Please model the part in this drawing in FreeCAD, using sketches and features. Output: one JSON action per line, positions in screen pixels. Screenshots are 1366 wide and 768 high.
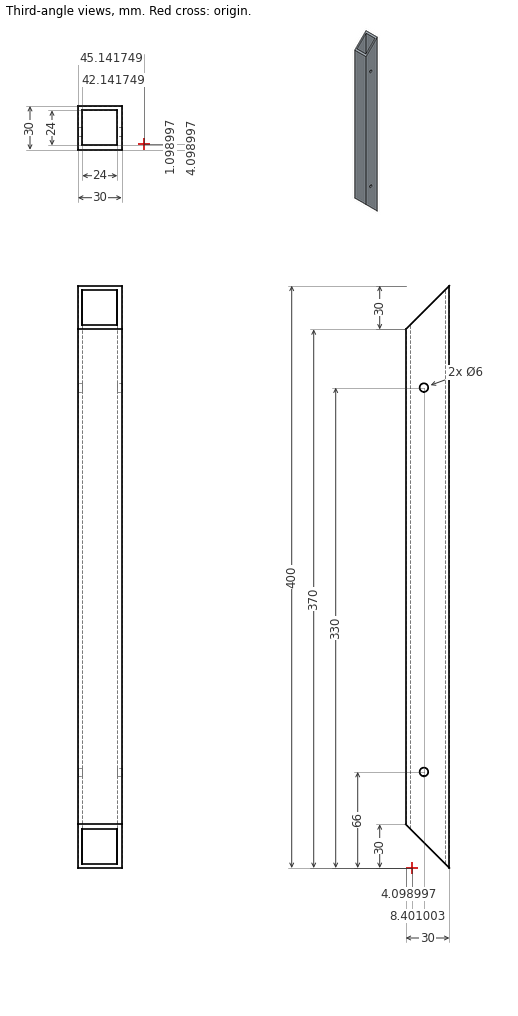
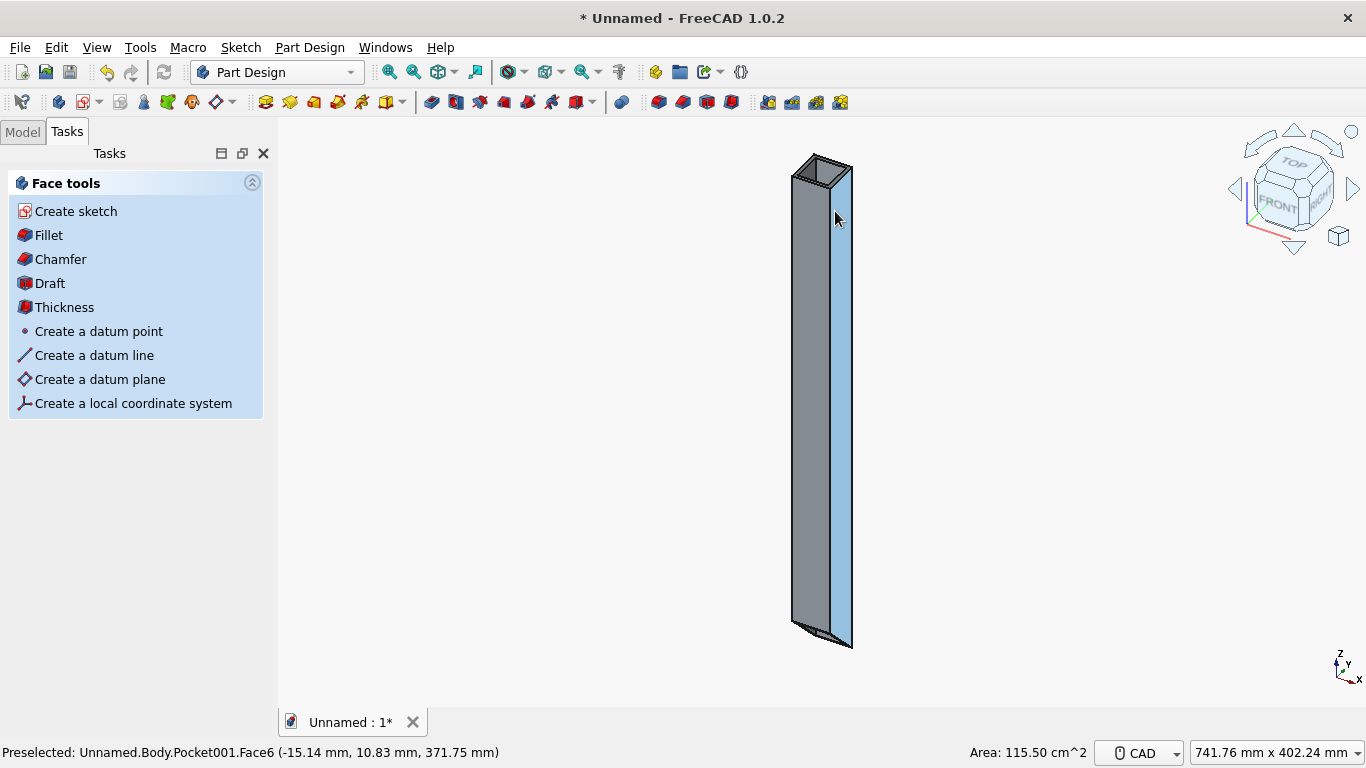
{"action": "left_click", "coordinate": [84, 102]}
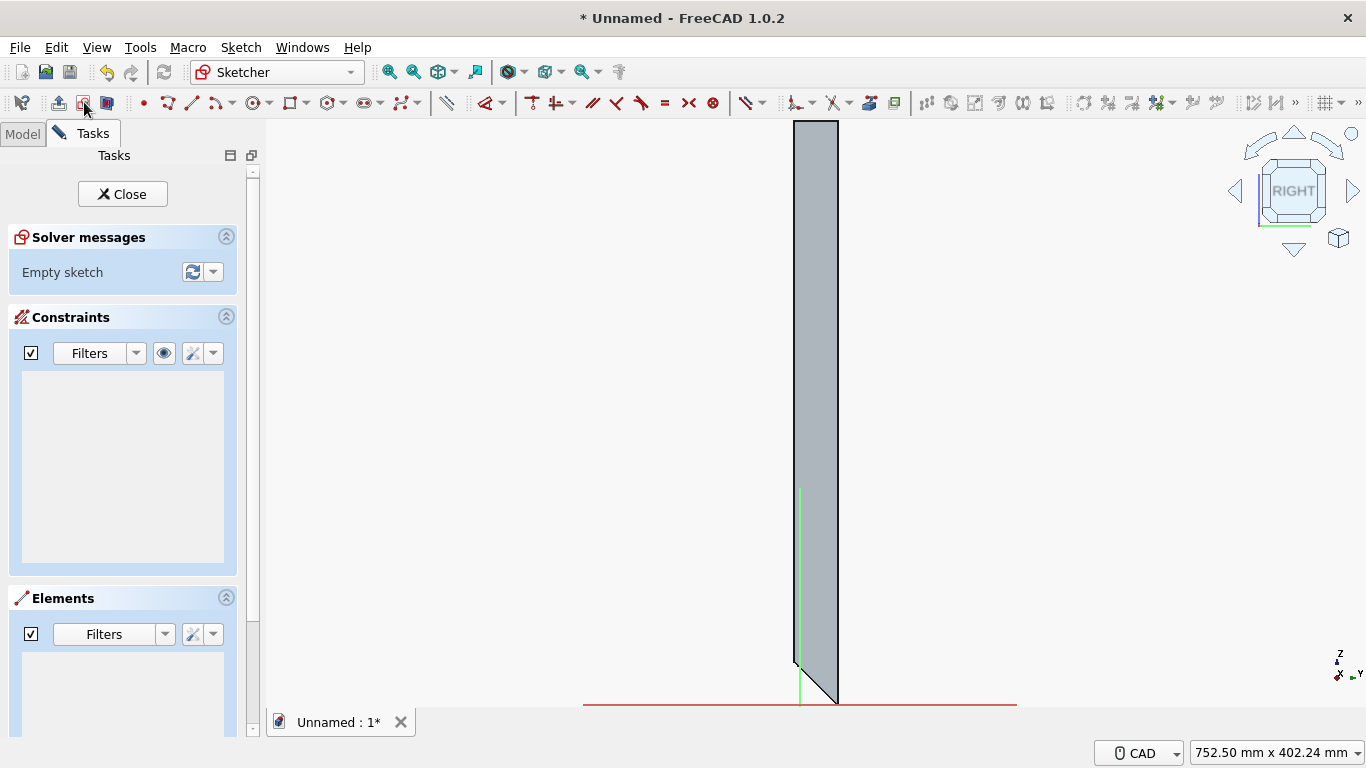
{"action": "scroll", "coordinate": [748, 413], "scroll_direction": "down", "scroll_amount": 5}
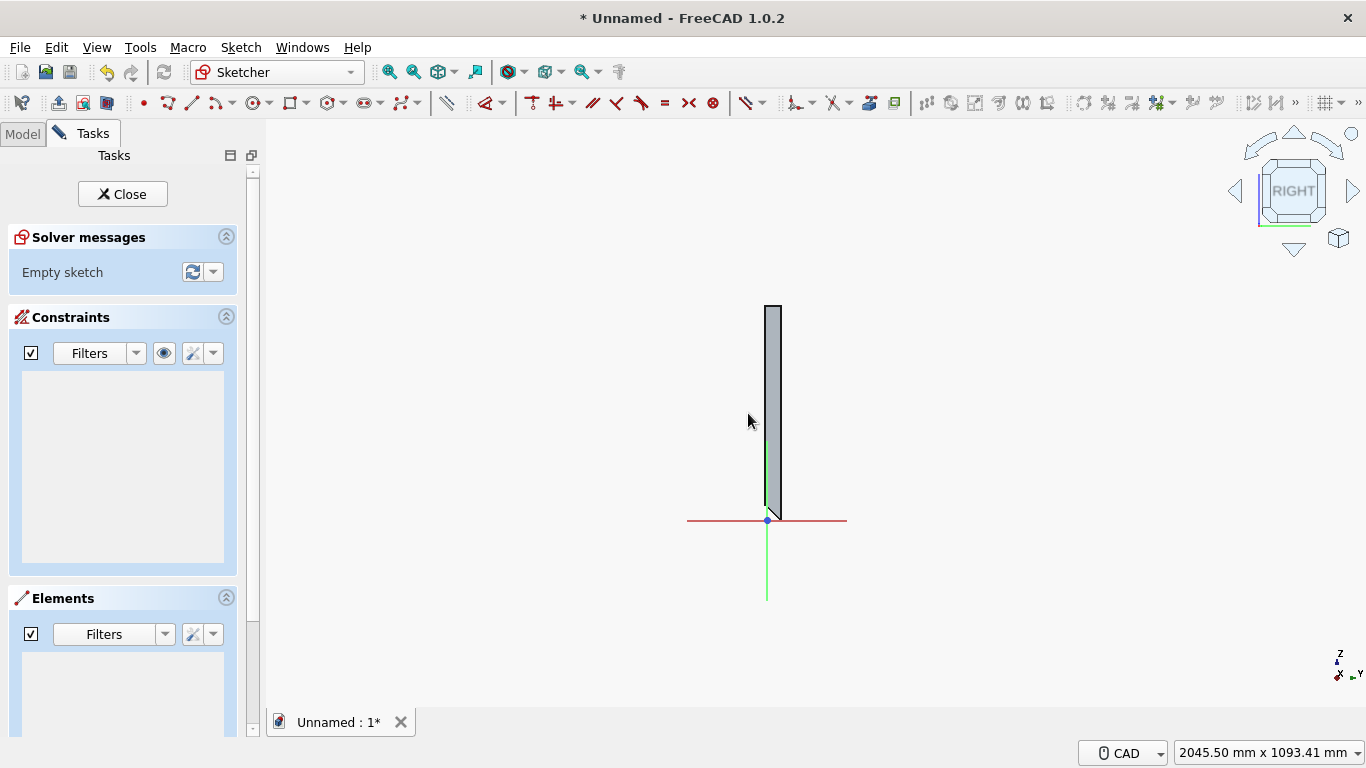
{"action": "scroll", "coordinate": [775, 309], "scroll_direction": "up", "scroll_amount": 15}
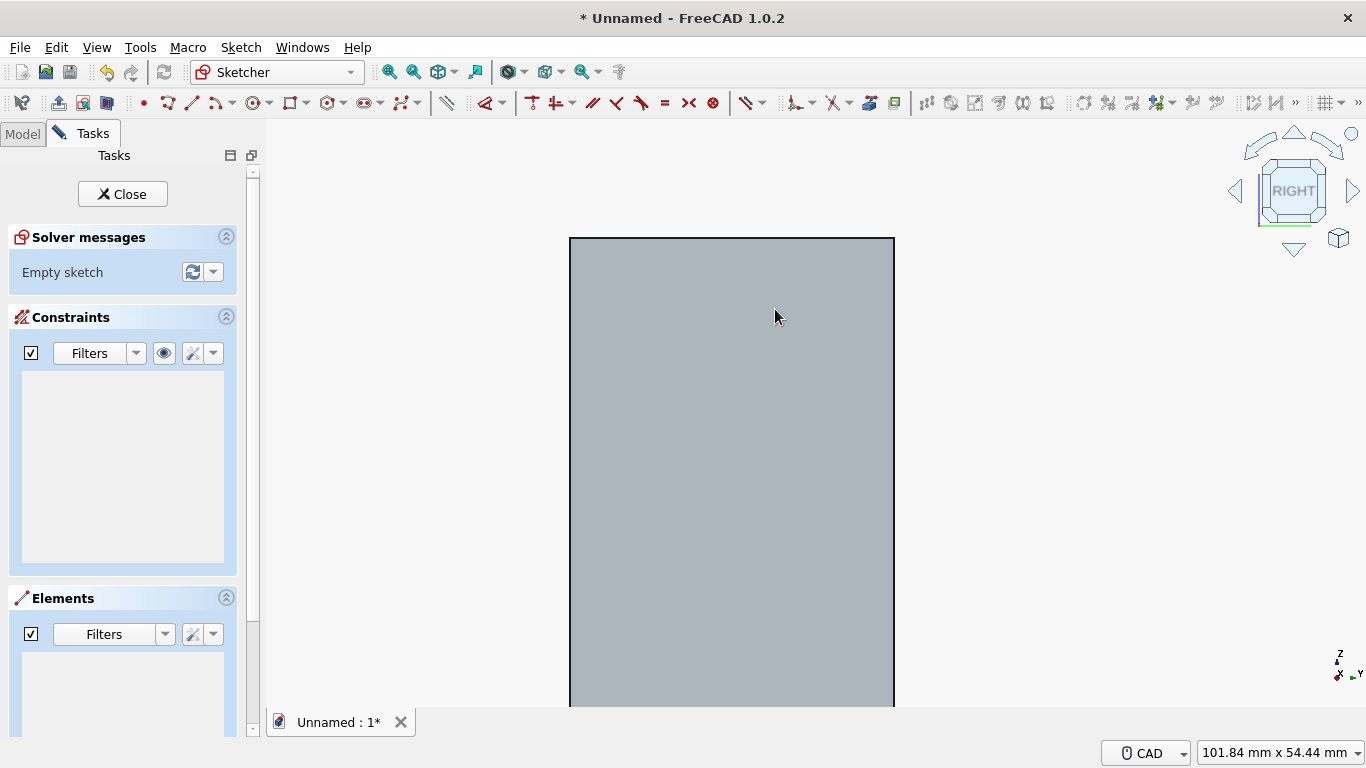
{"action": "left_click", "coordinate": [168, 104]}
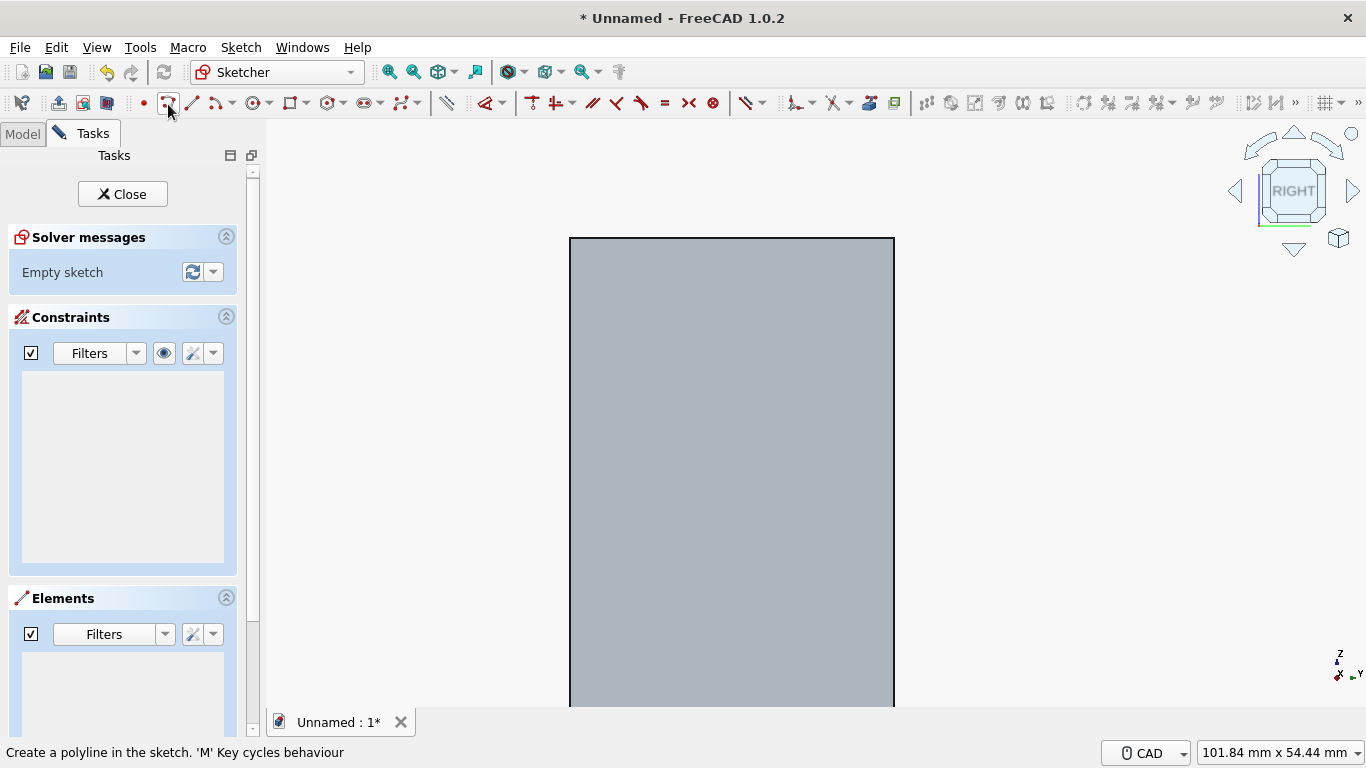
{"action": "left_click", "coordinate": [570, 562]}
{"action": "left_click", "coordinate": [894, 238]}
{"action": "left_click", "coordinate": [570, 238]}
{"action": "left_click", "coordinate": [570, 563]}
{"action": "key", "text": "Escape"}
{"action": "key", "text": "Escape"}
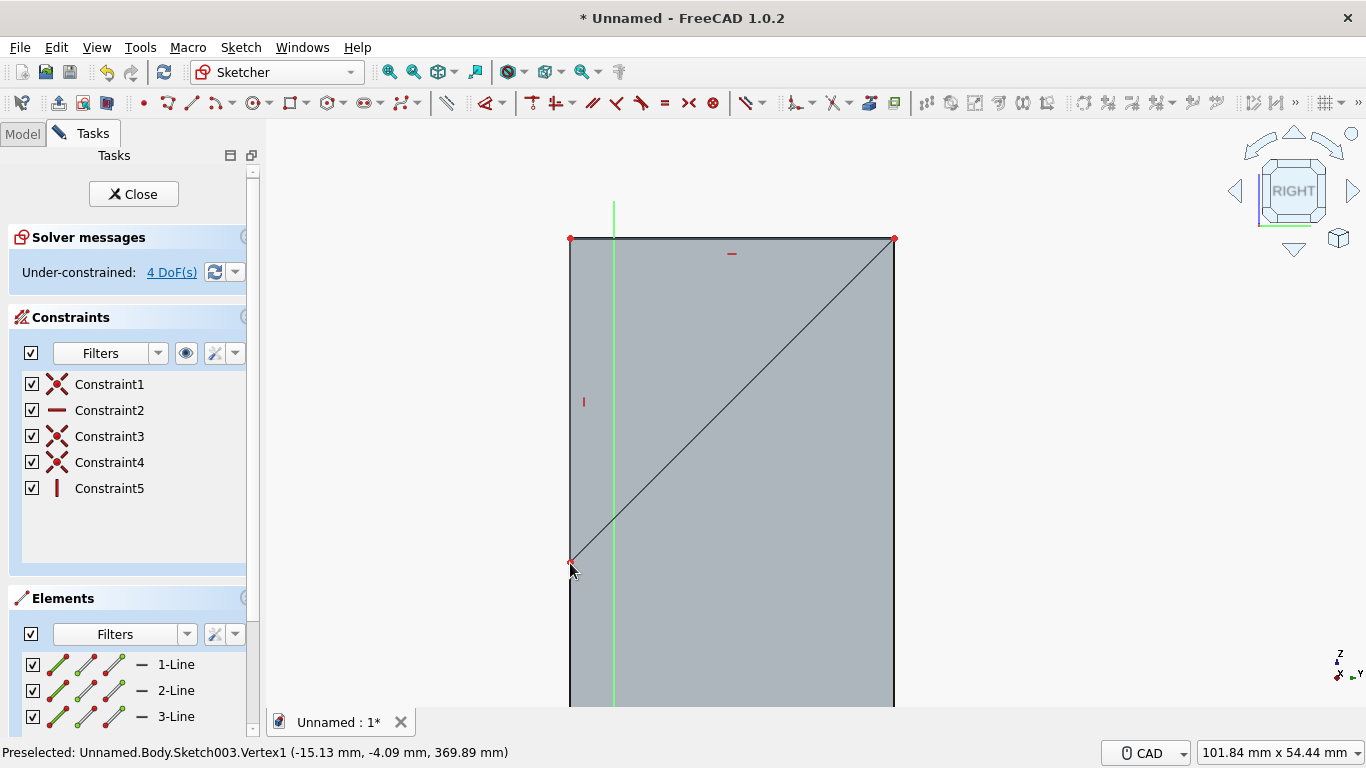
{"action": "key", "text": "d"}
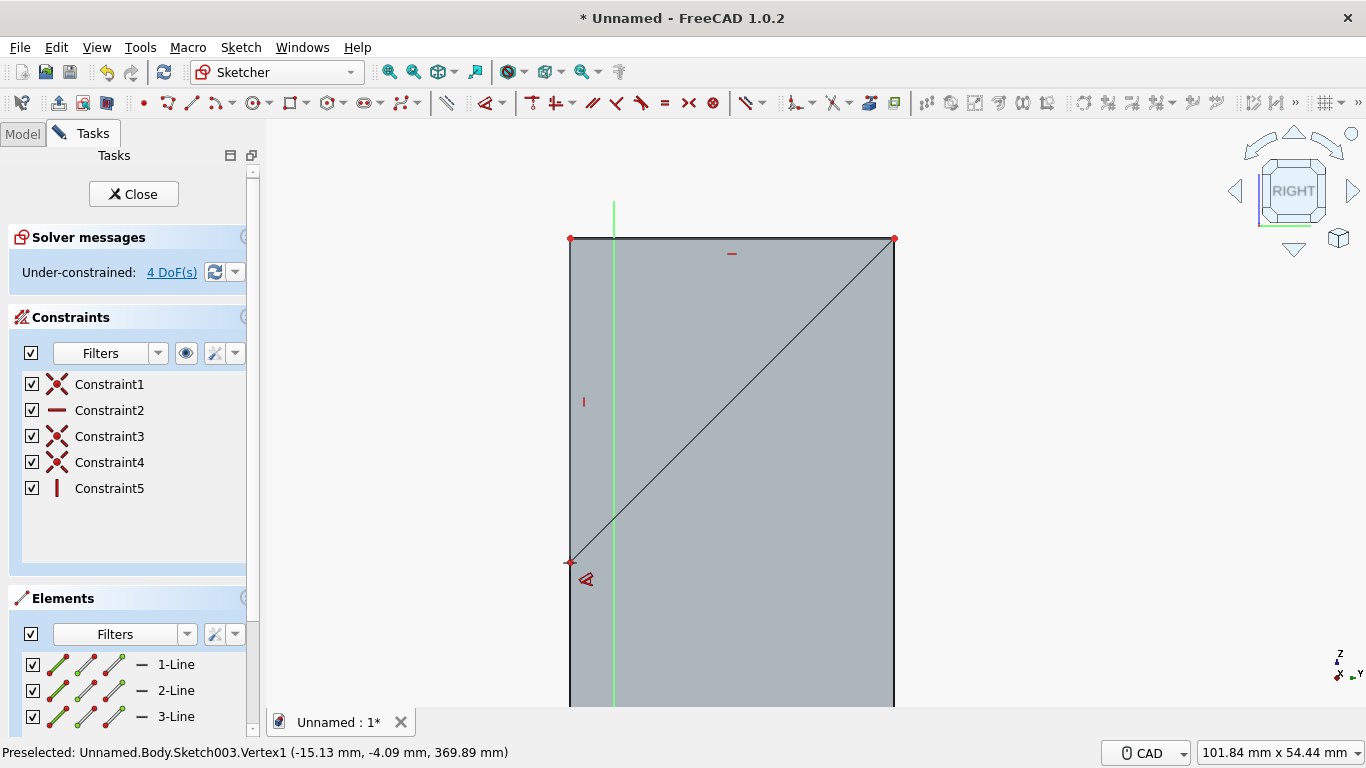
{"action": "left_click", "coordinate": [797, 239]}
{"action": "left_click", "coordinate": [732, 205]}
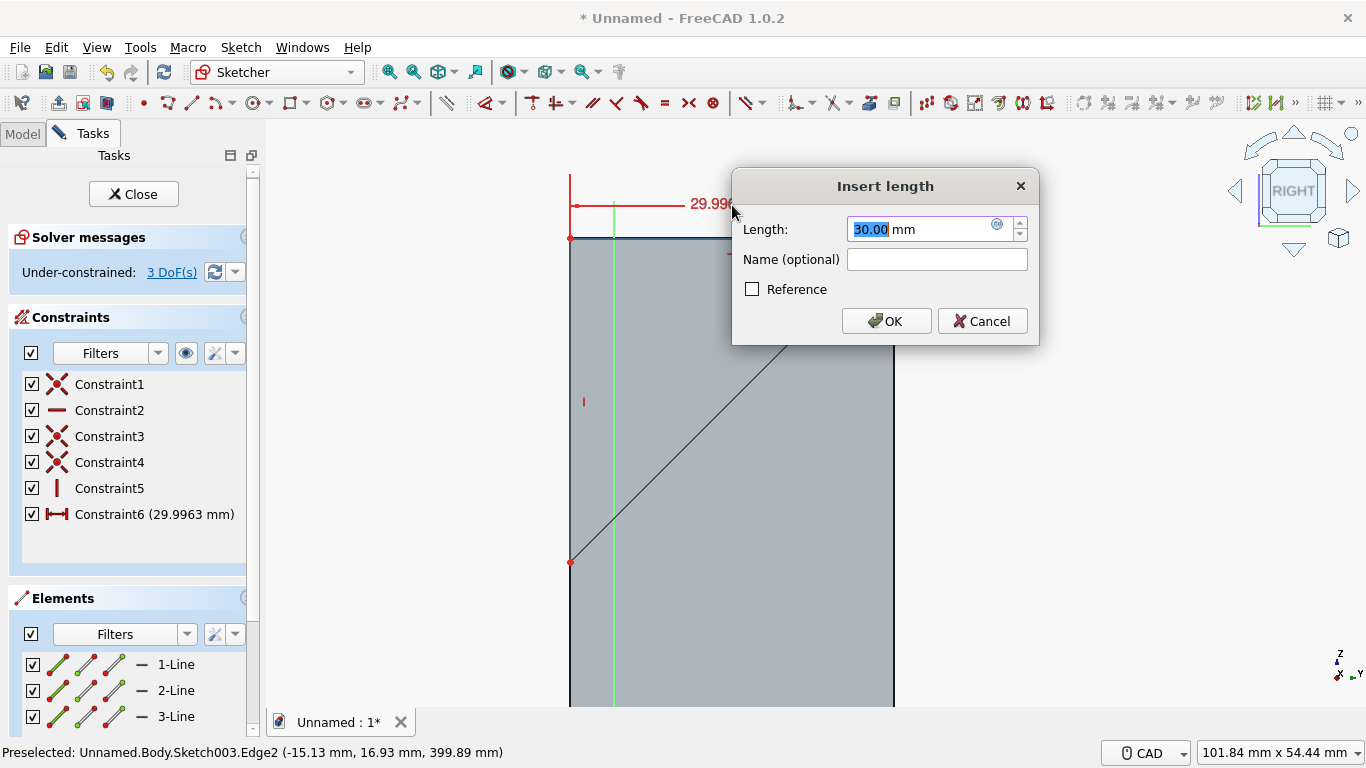
{"action": "type", "text": "30"}
{"action": "key", "text": "Return"}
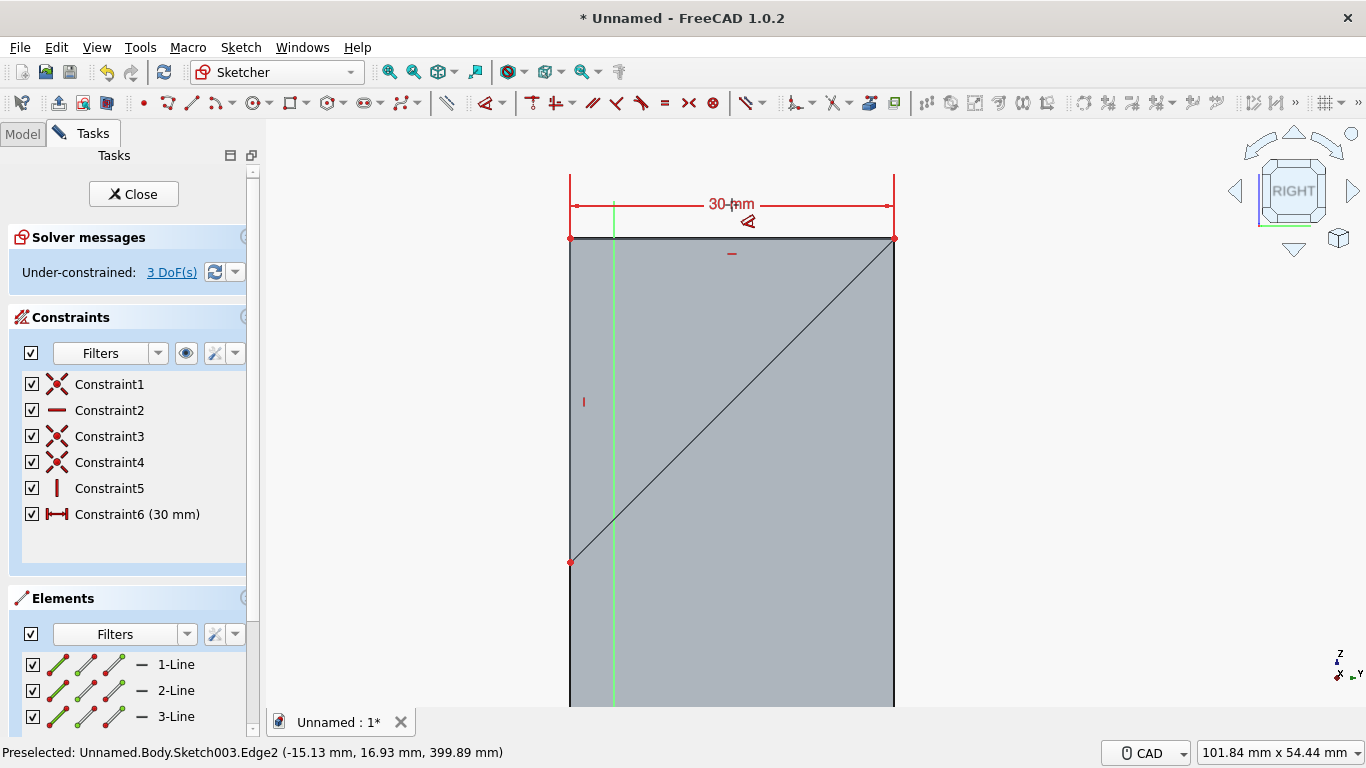
{"action": "left_click", "coordinate": [570, 336]}
{"action": "left_click", "coordinate": [536, 401]}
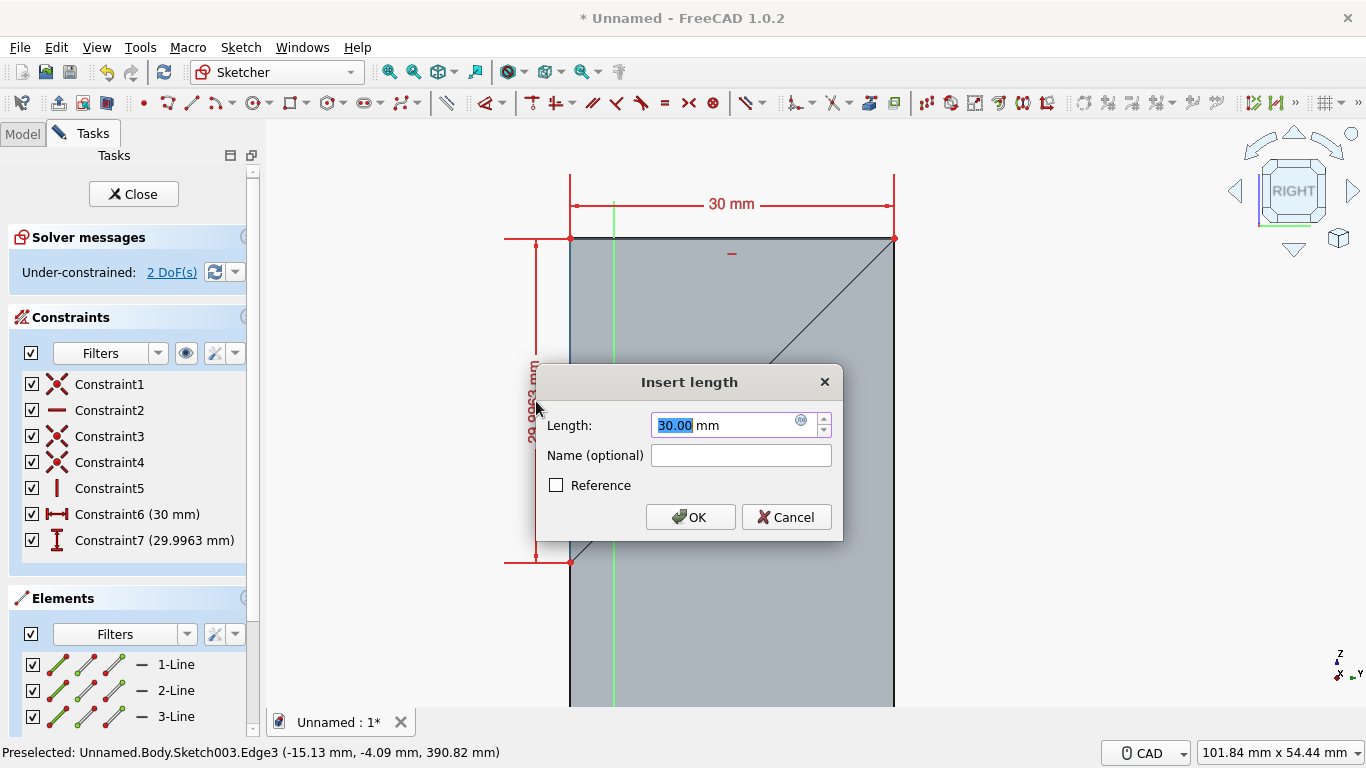
{"action": "type", "text": "30"}
{"action": "key", "text": "Return"}